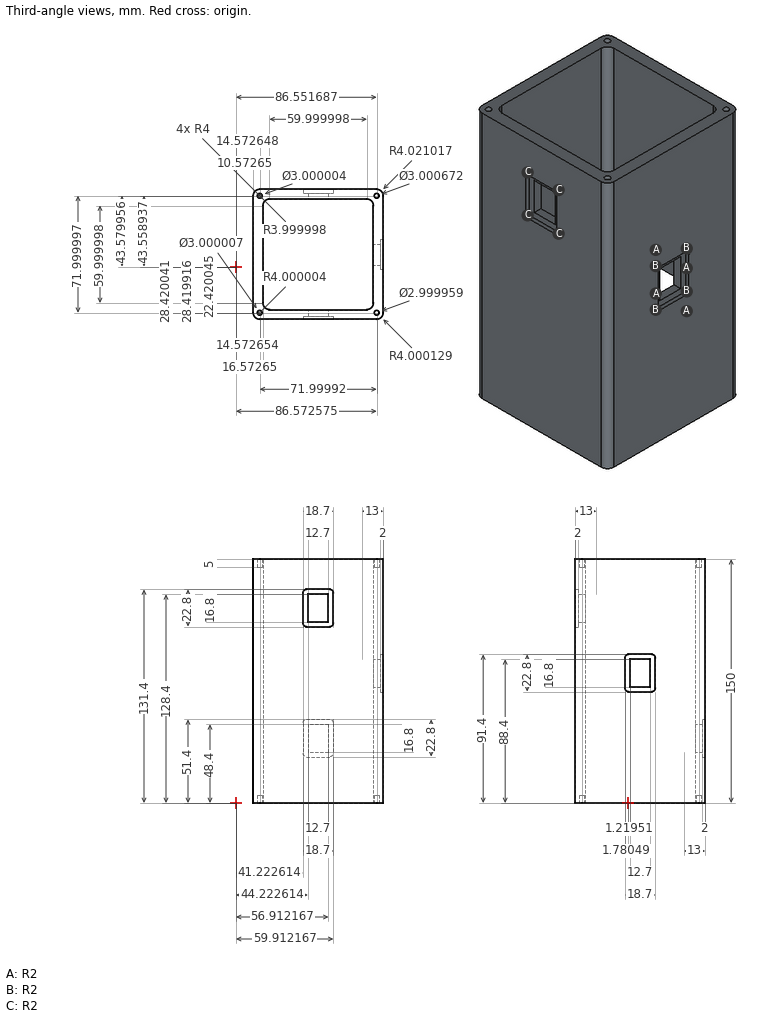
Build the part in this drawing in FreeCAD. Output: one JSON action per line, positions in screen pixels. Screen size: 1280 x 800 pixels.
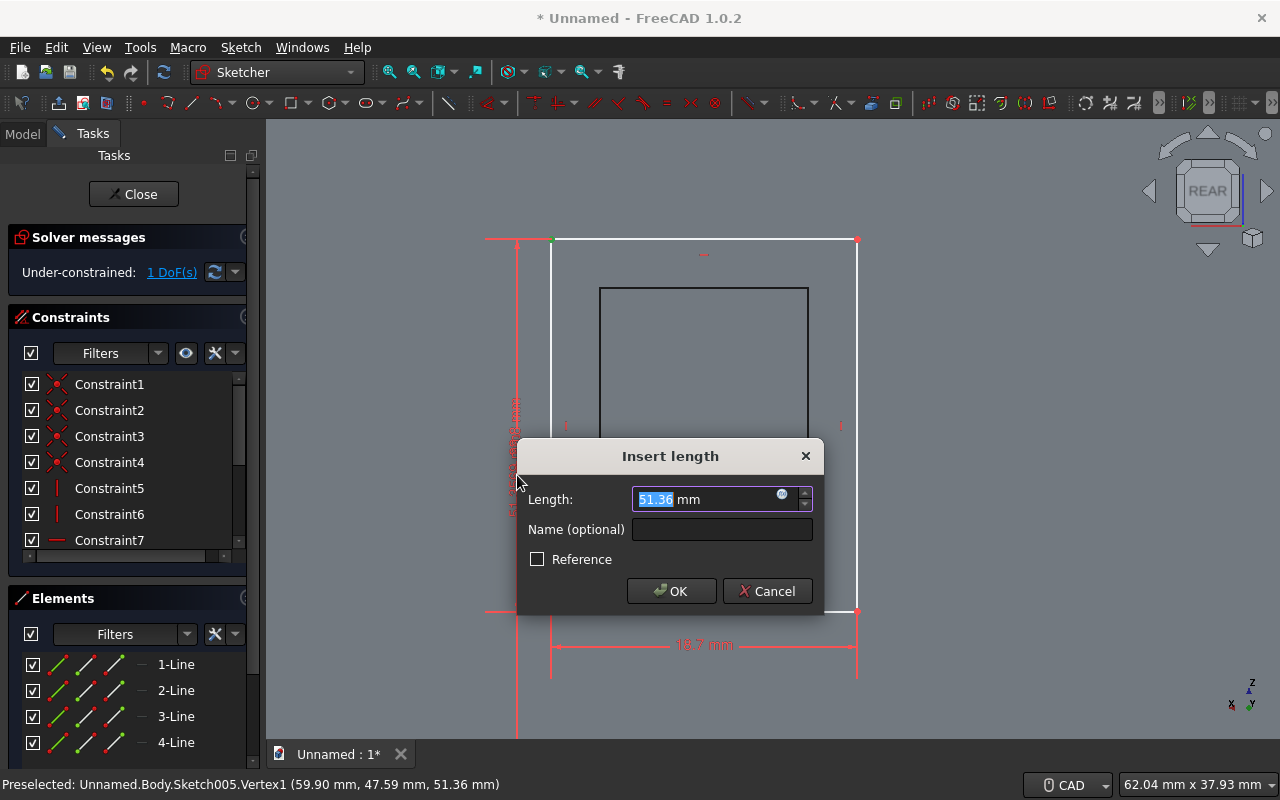
{"action": "type", "text": "51.4"}
{"action": "key", "text": "Return"}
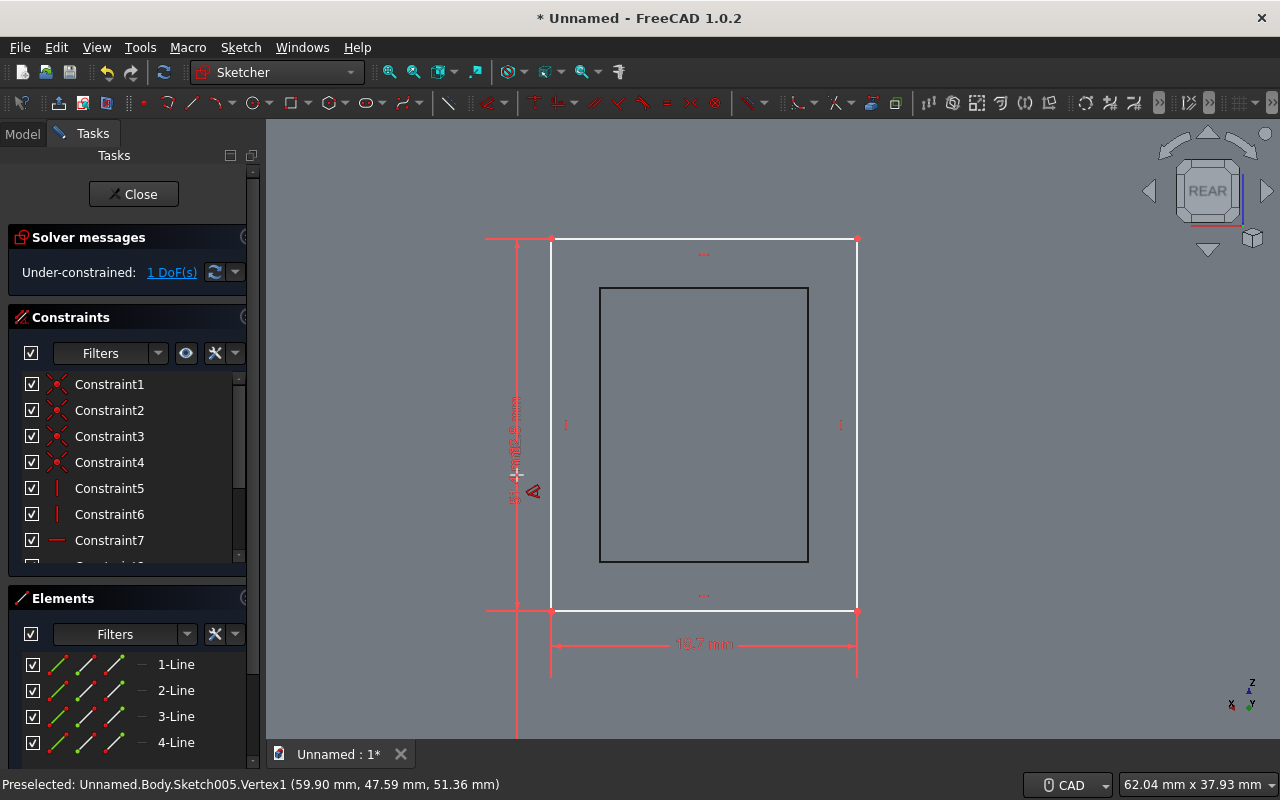
{"action": "left_click", "coordinate": [551, 239]}
{"action": "left_click", "coordinate": [833, 205]}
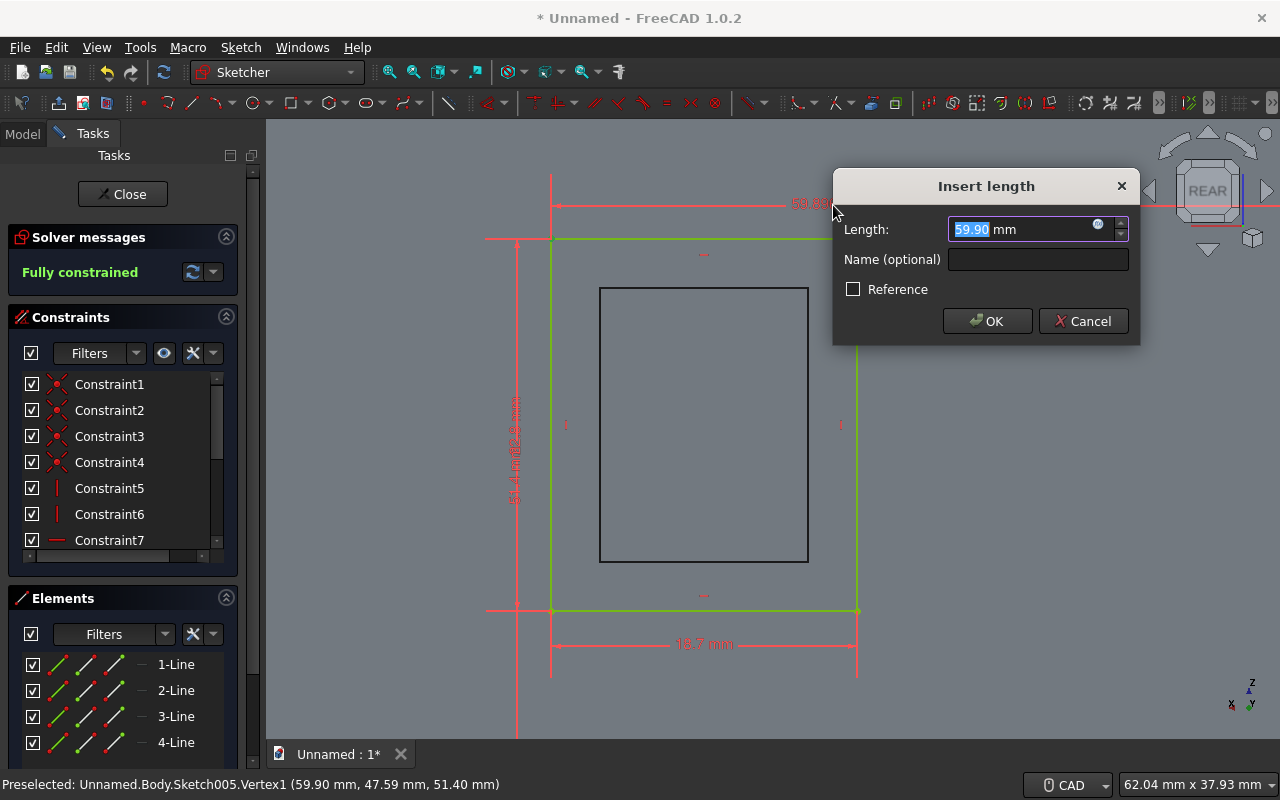
{"action": "type", "text": "59.912167"}
{"action": "key", "text": "Return"}
{"action": "key", "text": "Escape"}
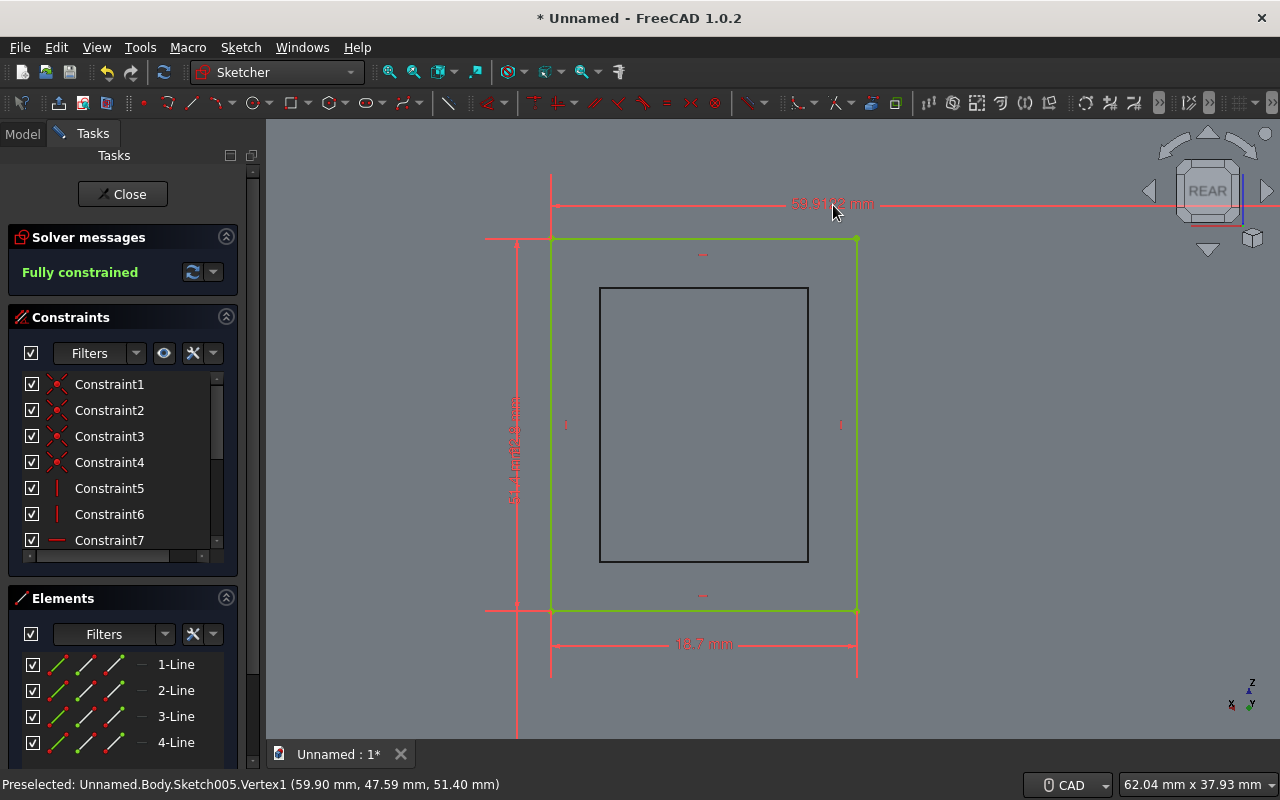
{"action": "left_click", "coordinate": [123, 194]}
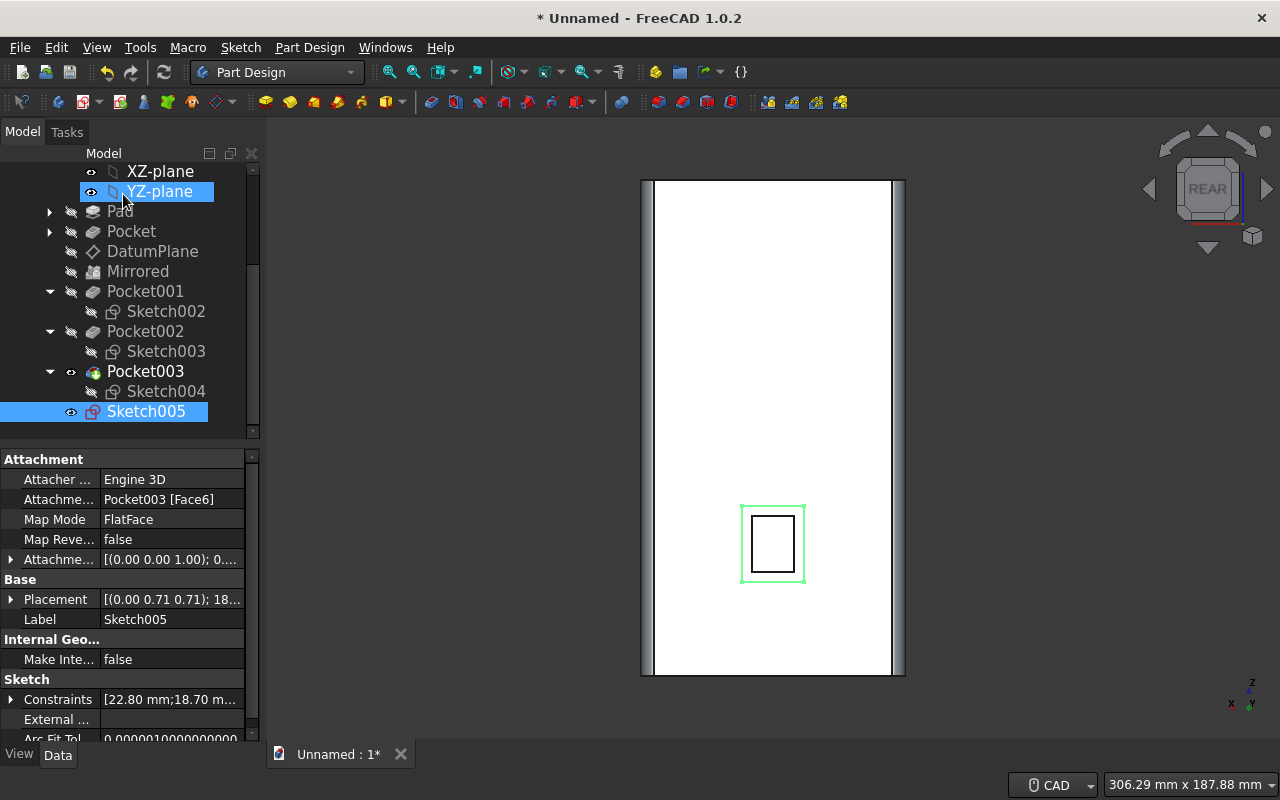
{"action": "left_click", "coordinate": [432, 102]}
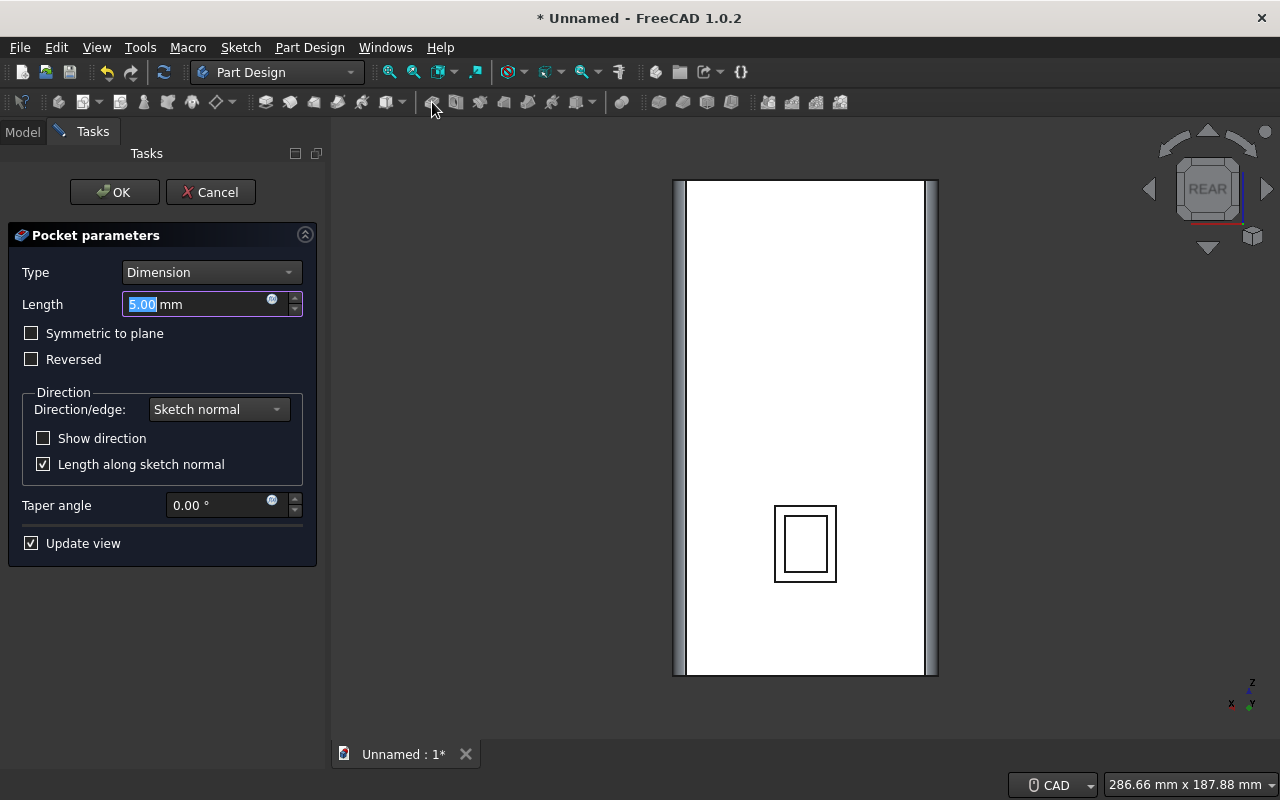
{"action": "type", "text": "2"}
{"action": "key", "text": "Tab"}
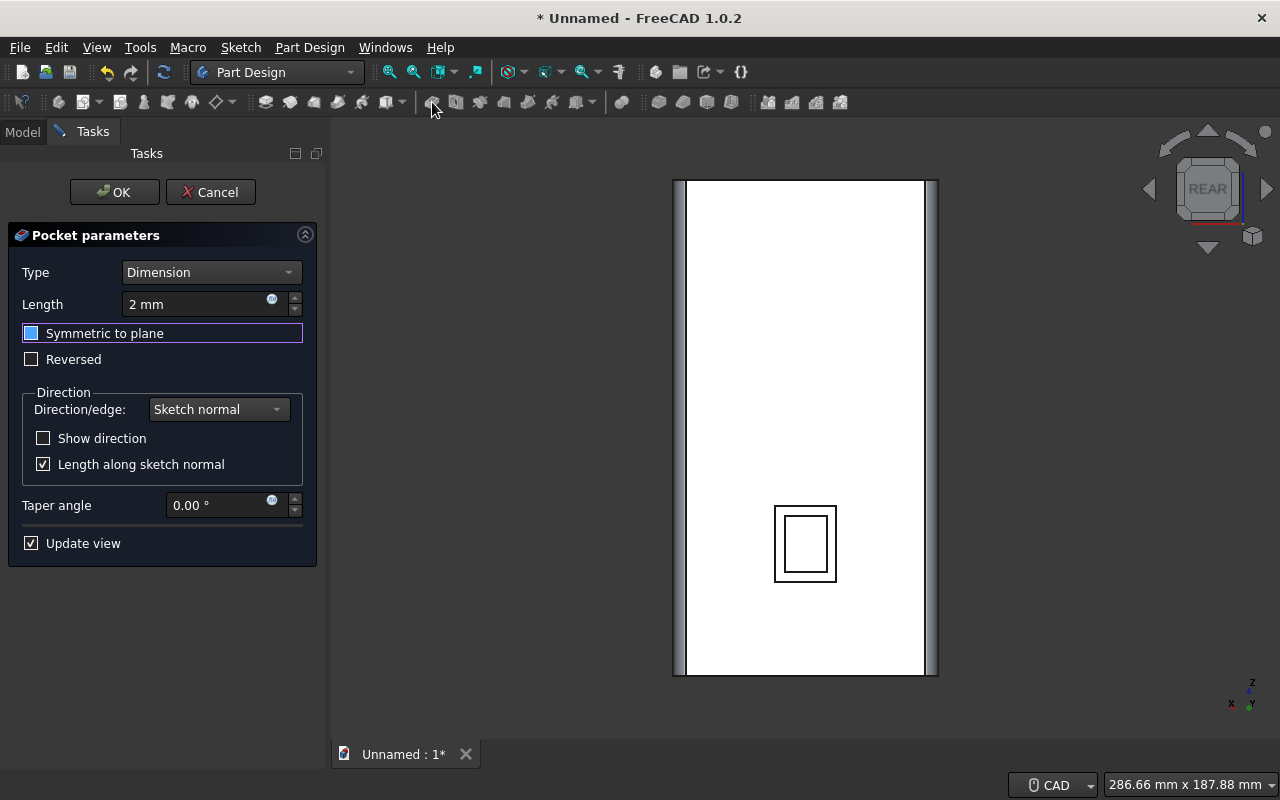
{"action": "left_click", "coordinate": [115, 192]}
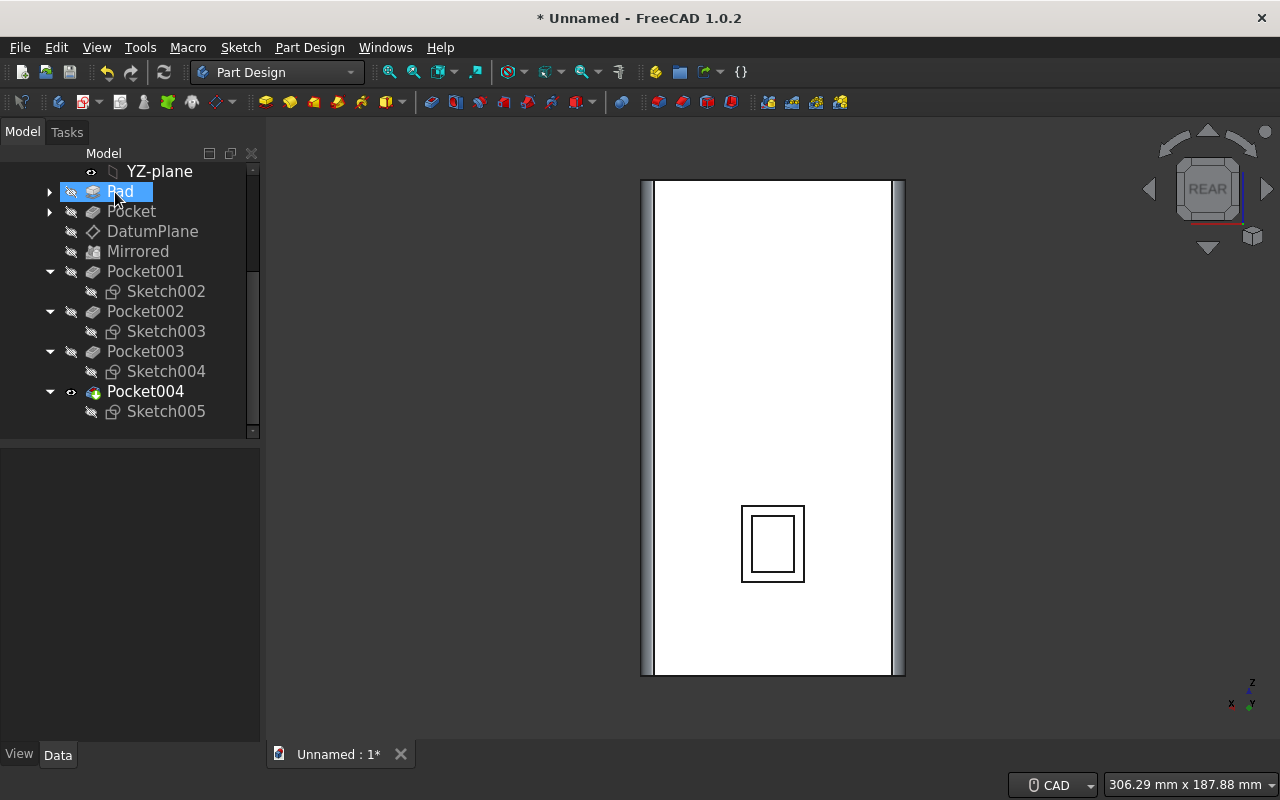
{"action": "scroll", "coordinate": [742, 581], "scroll_direction": "up", "scroll_amount": 9}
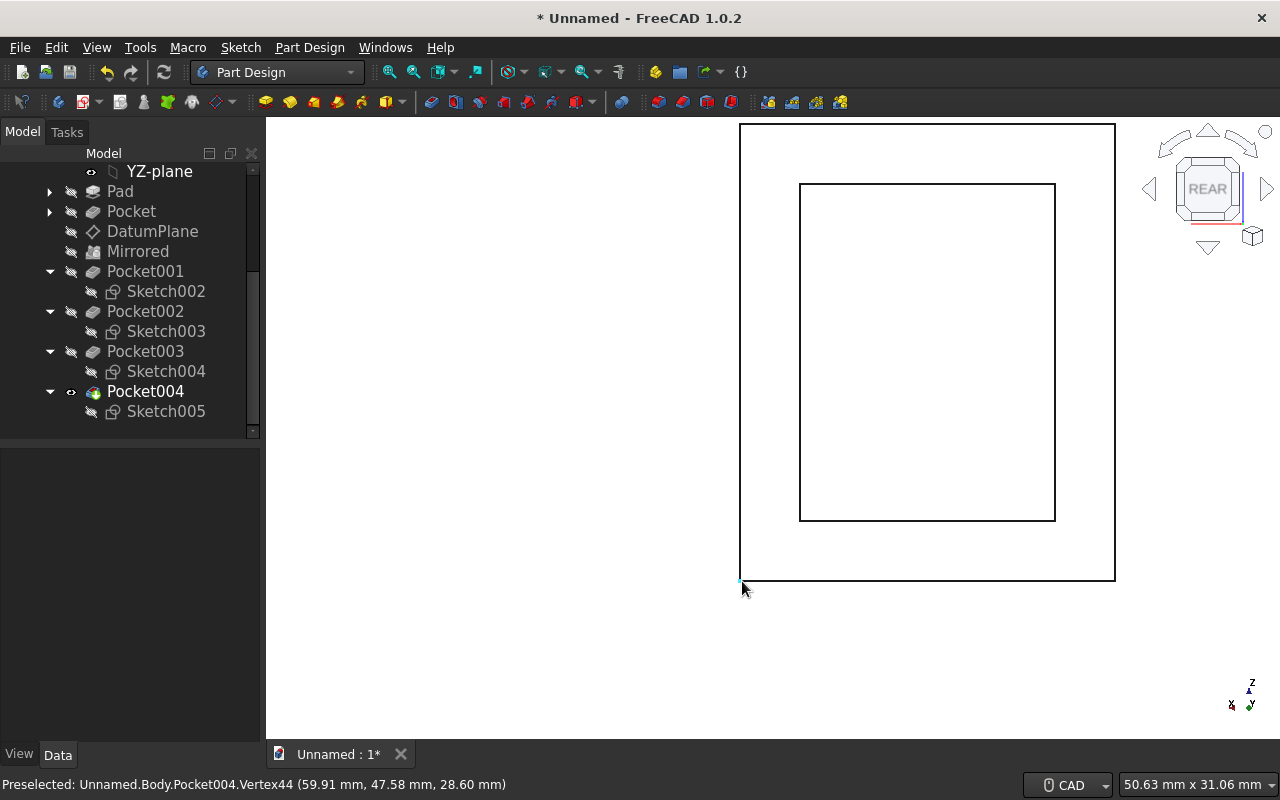
{"action": "left_click", "coordinate": [390, 72]}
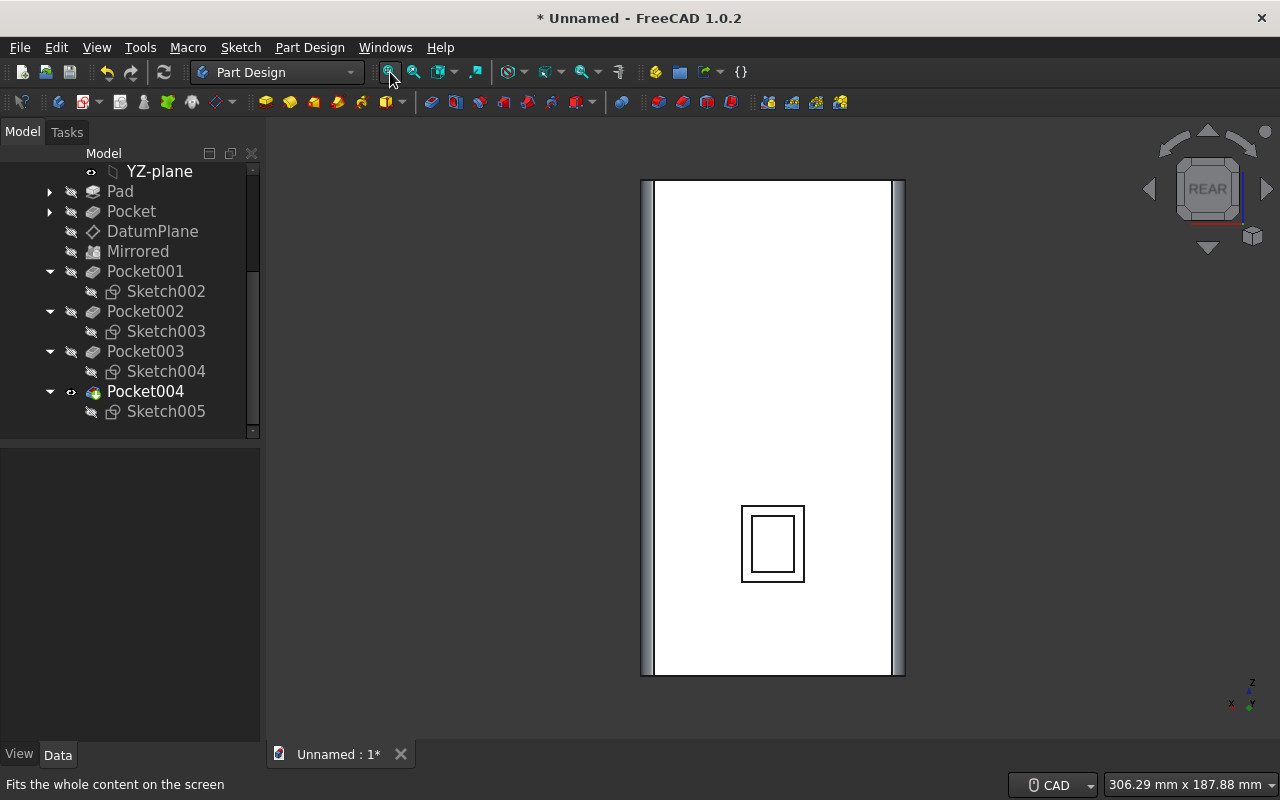
{"action": "key", "text": "0"}